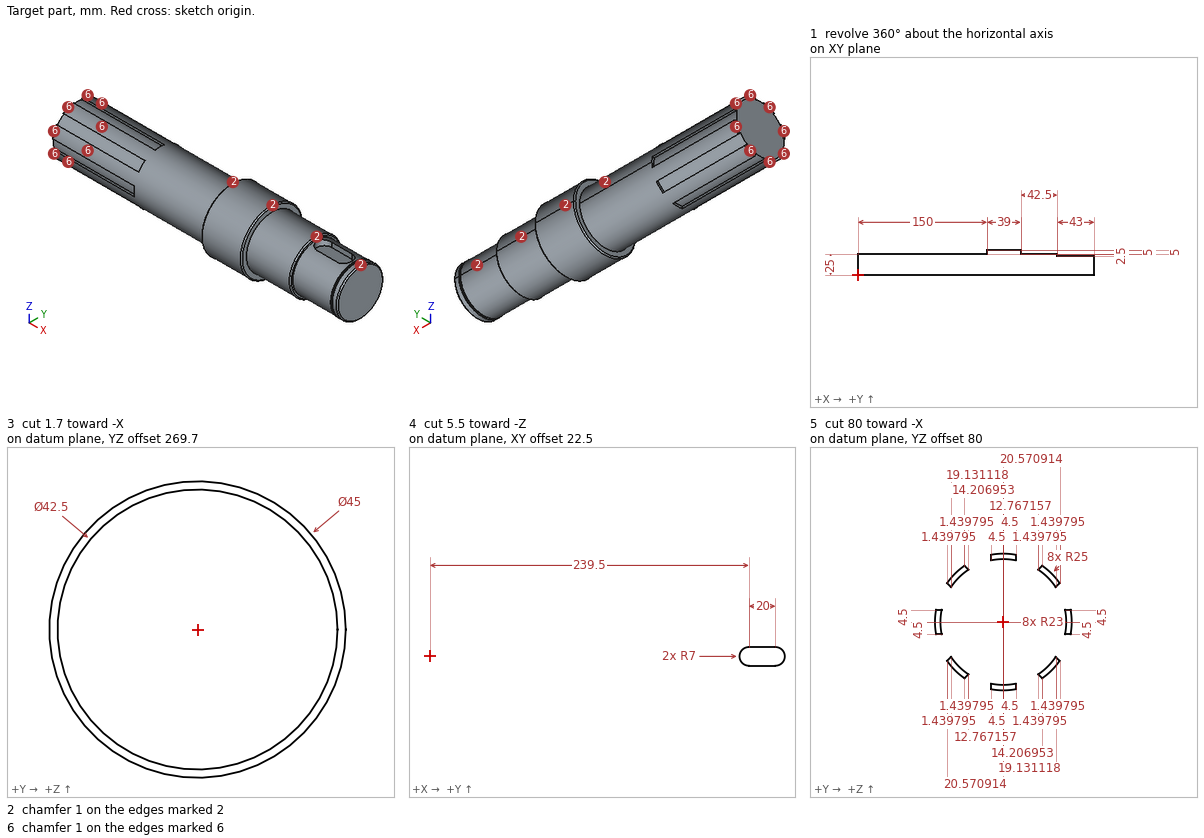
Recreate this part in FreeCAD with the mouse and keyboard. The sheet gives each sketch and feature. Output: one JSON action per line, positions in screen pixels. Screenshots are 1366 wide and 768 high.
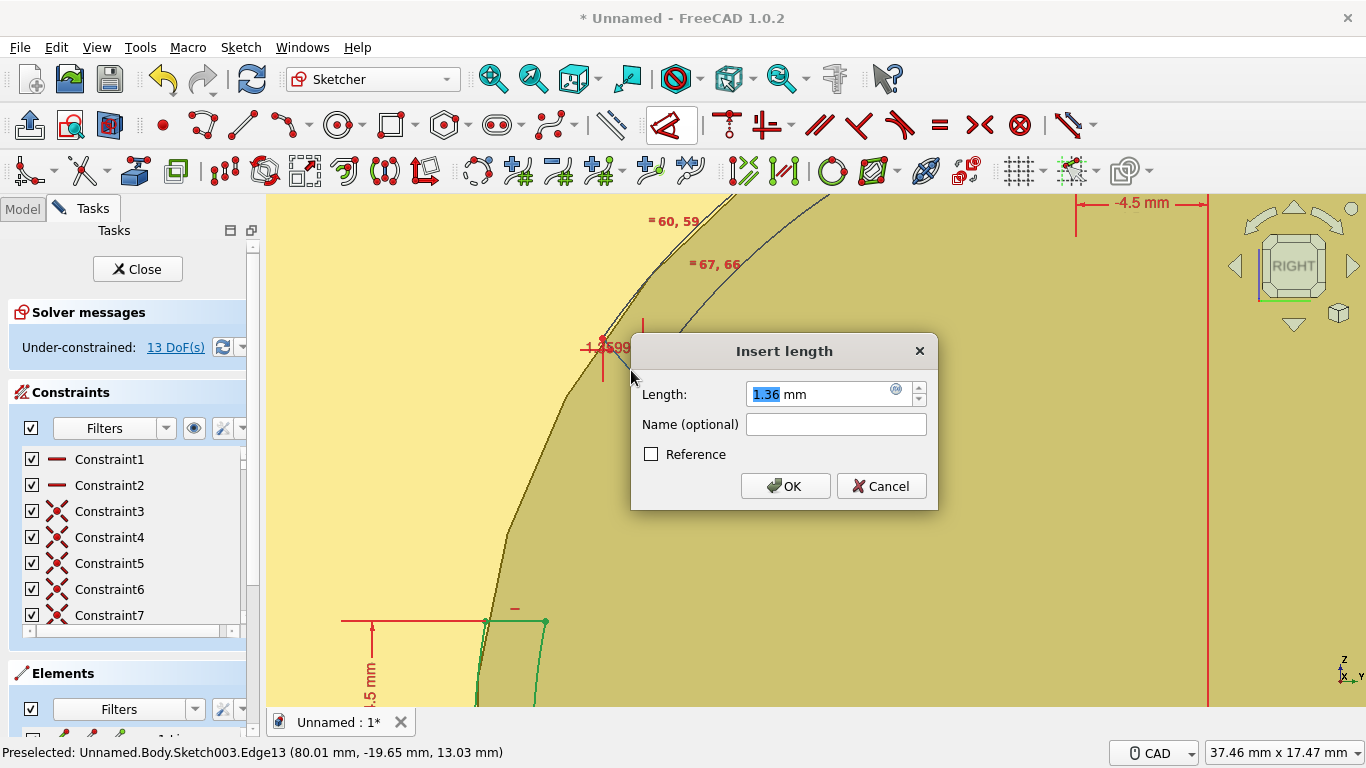
{"action": "type", "text": "1.439795"}
{"action": "key", "text": "Return"}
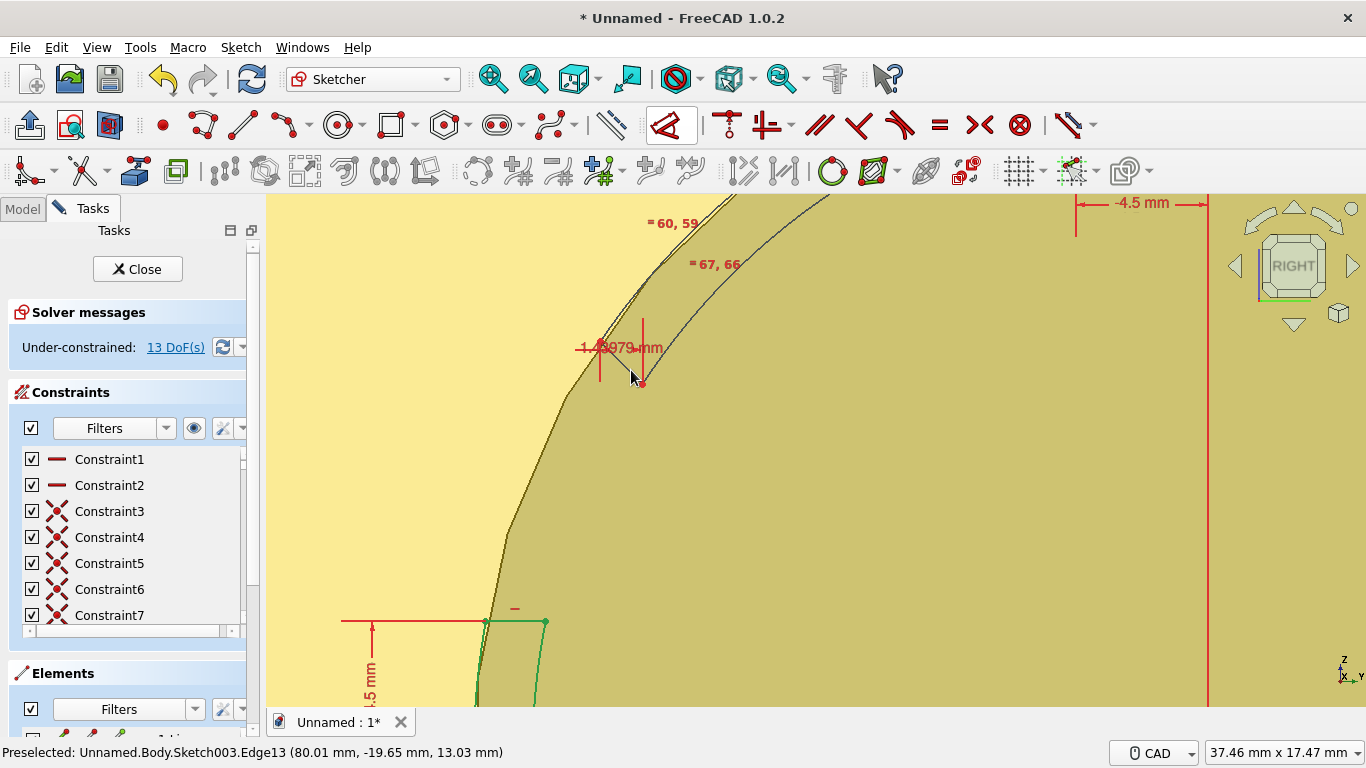
{"action": "scroll", "coordinate": [631, 374], "scroll_direction": "down", "scroll_amount": 8}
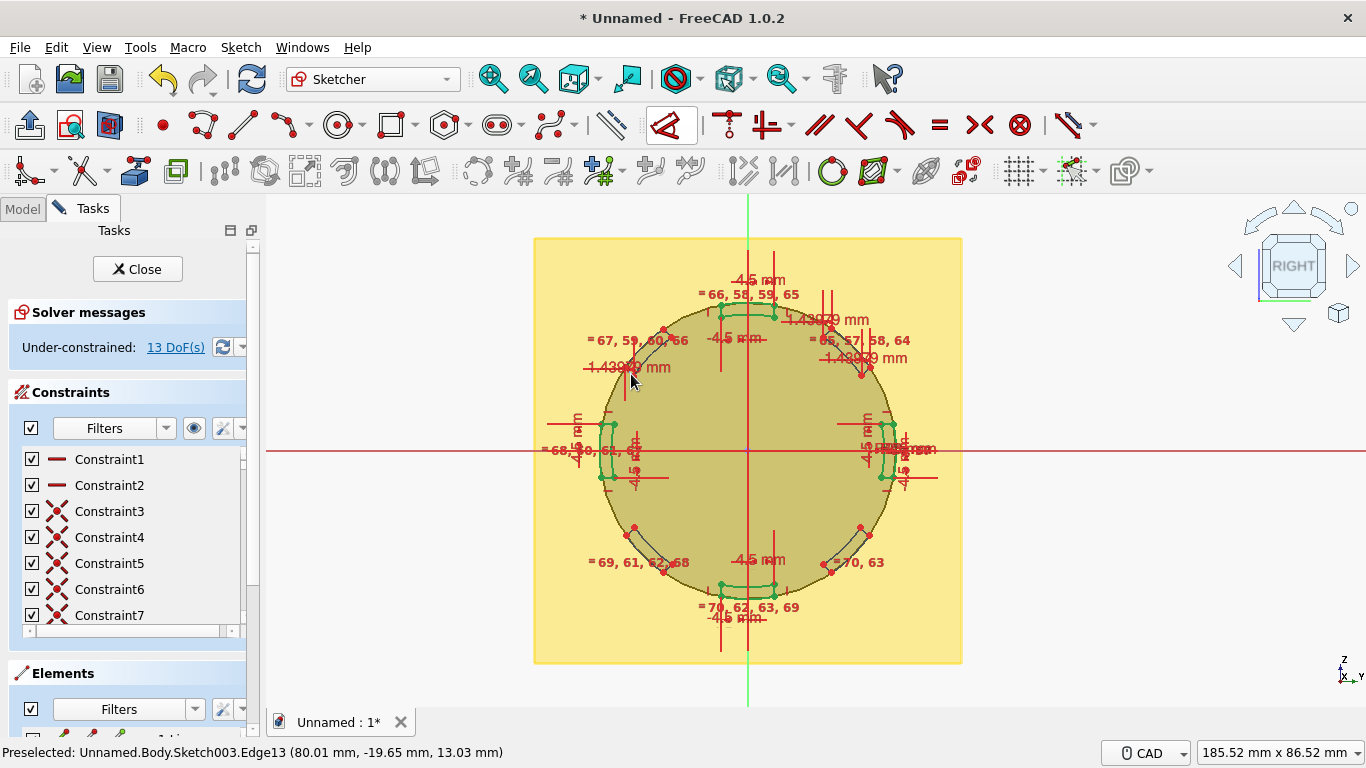
{"action": "scroll", "coordinate": [666, 332], "scroll_direction": "up", "scroll_amount": 8}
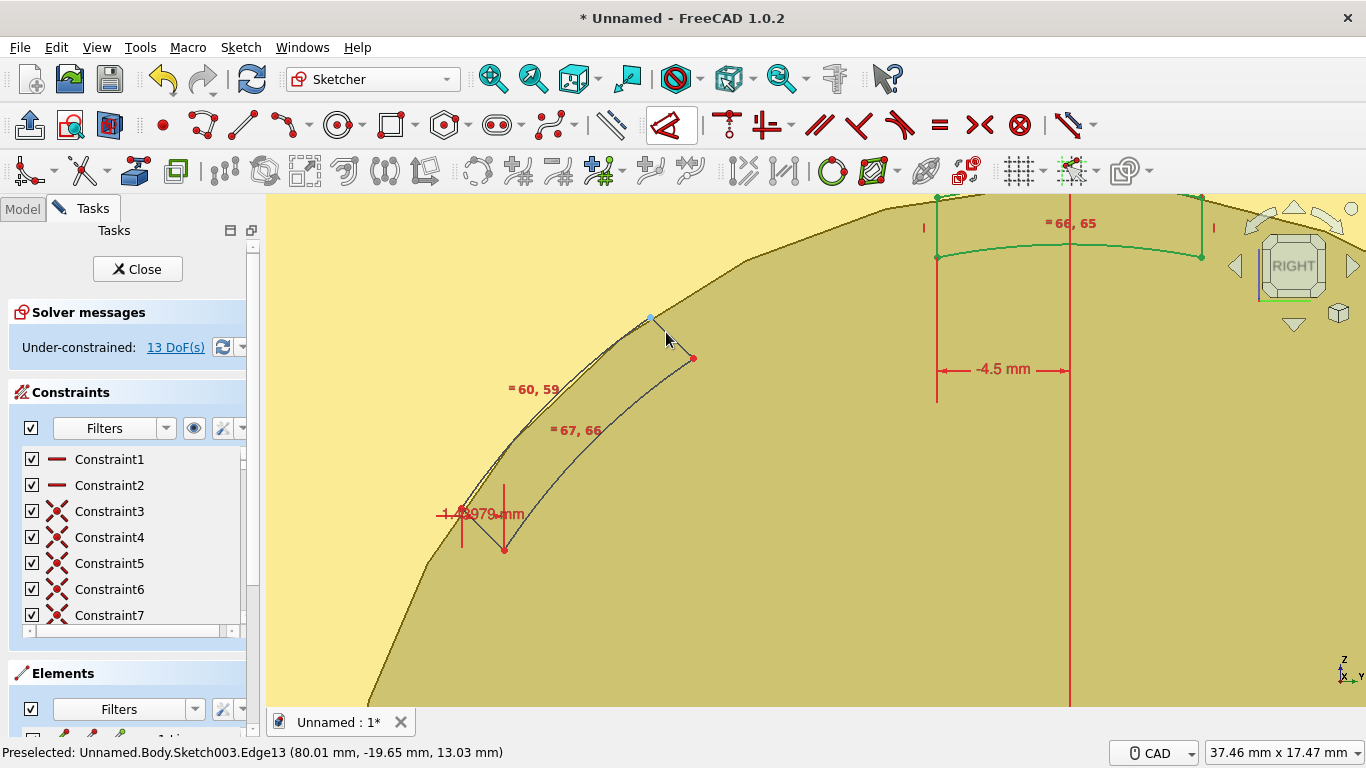
{"action": "left_click", "coordinate": [663, 330]}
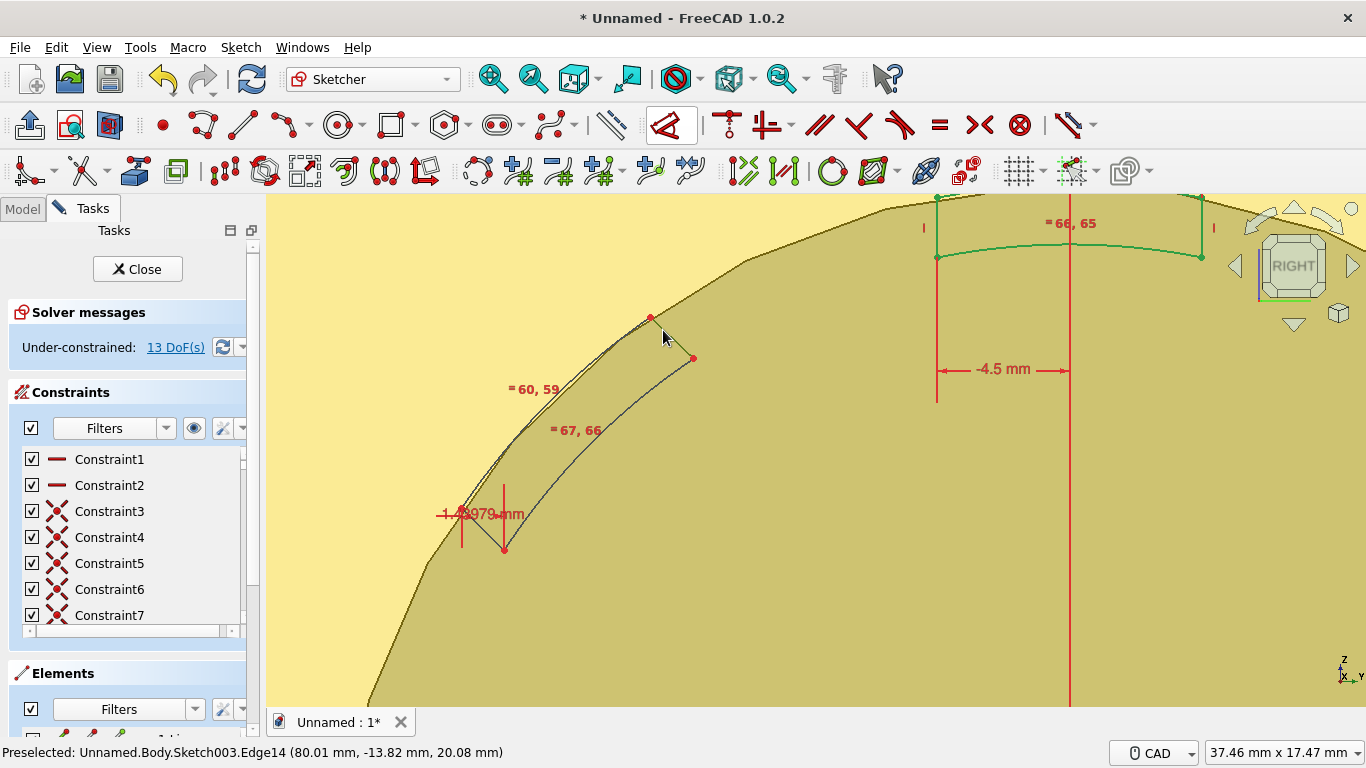
{"action": "key", "text": "l"}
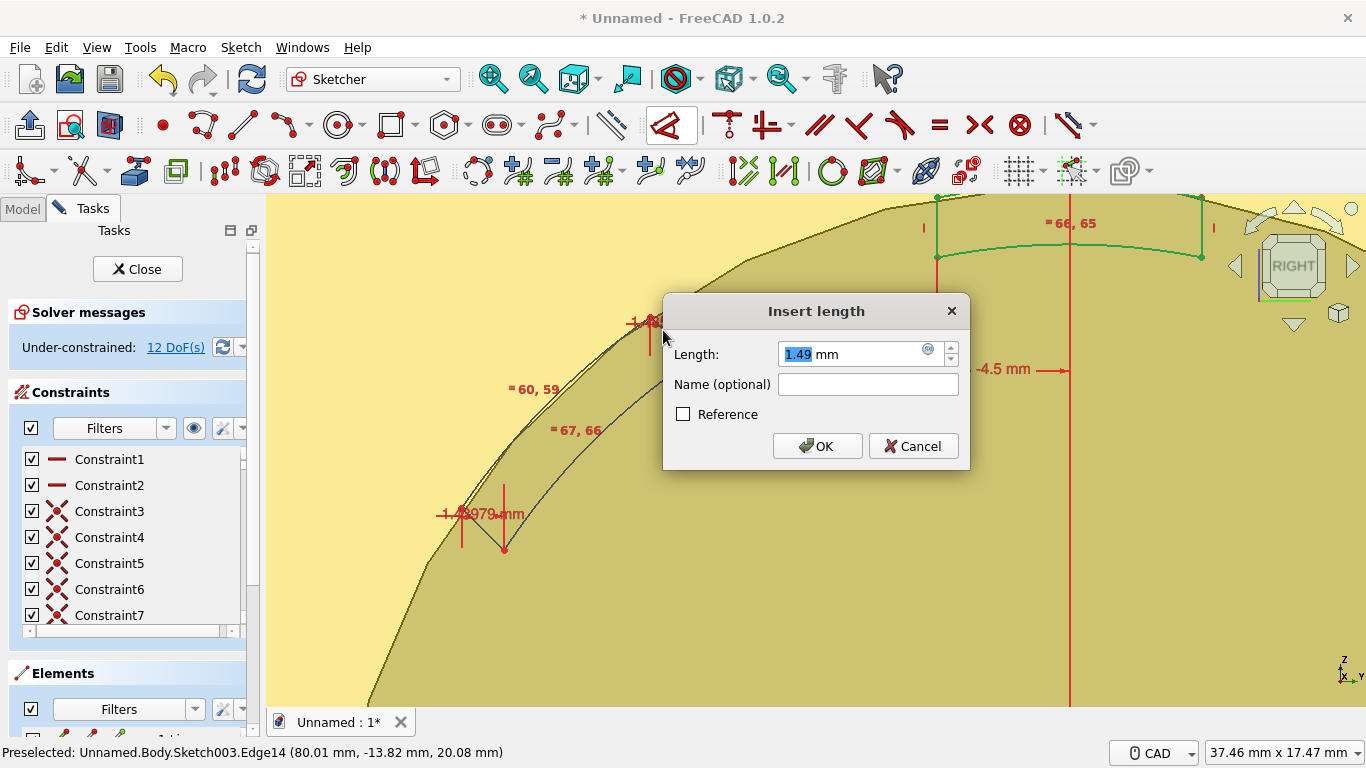
{"action": "type", "text": "1.439795"}
{"action": "key", "text": "Return"}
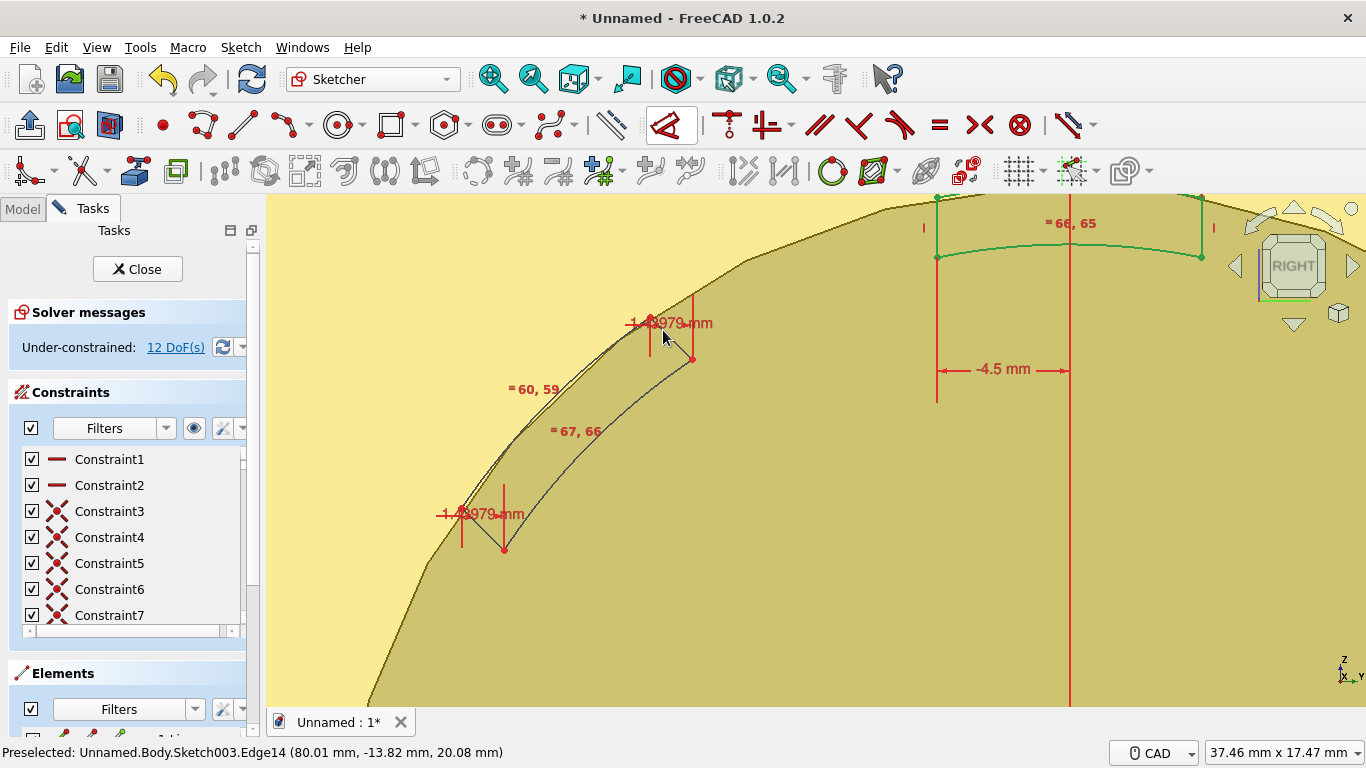
{"action": "scroll", "coordinate": [666, 332], "scroll_direction": "down", "scroll_amount": 8}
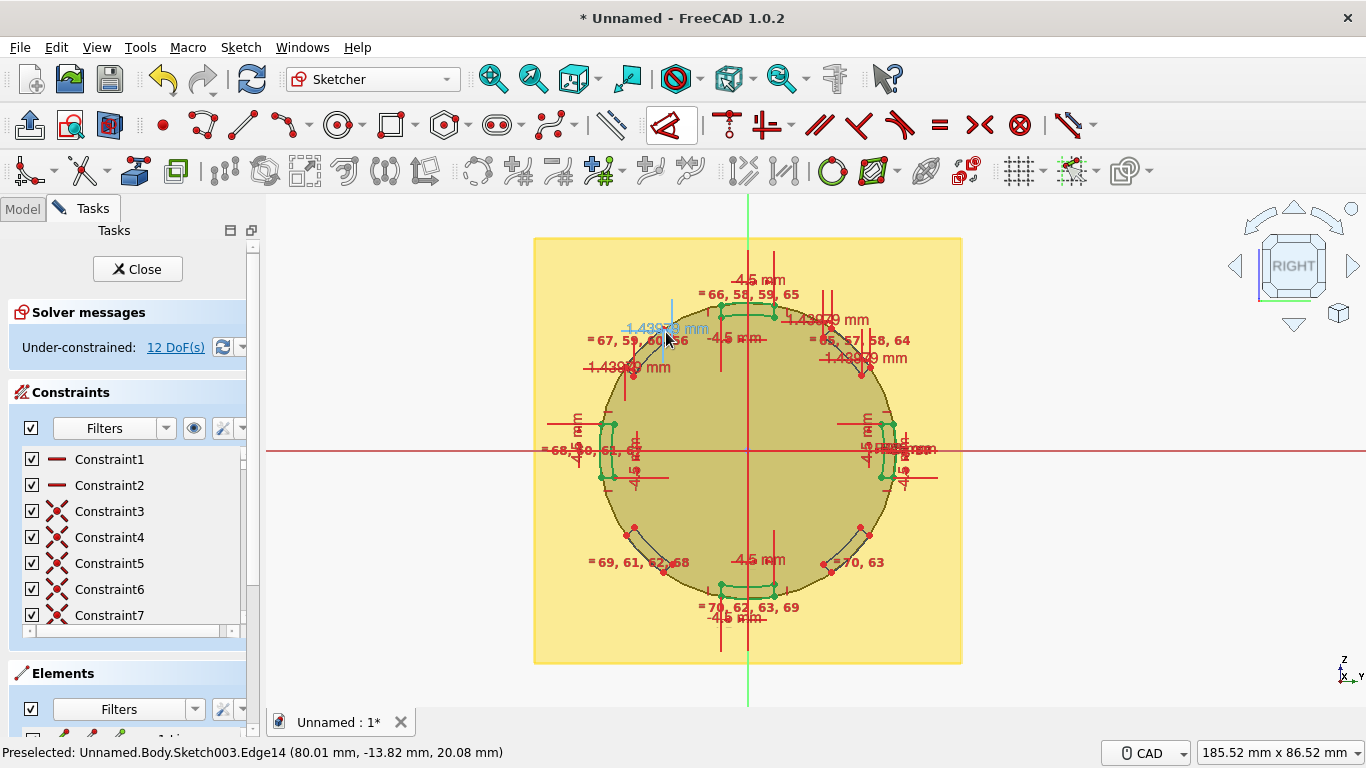
{"action": "scroll", "coordinate": [669, 567], "scroll_direction": "up", "scroll_amount": 8}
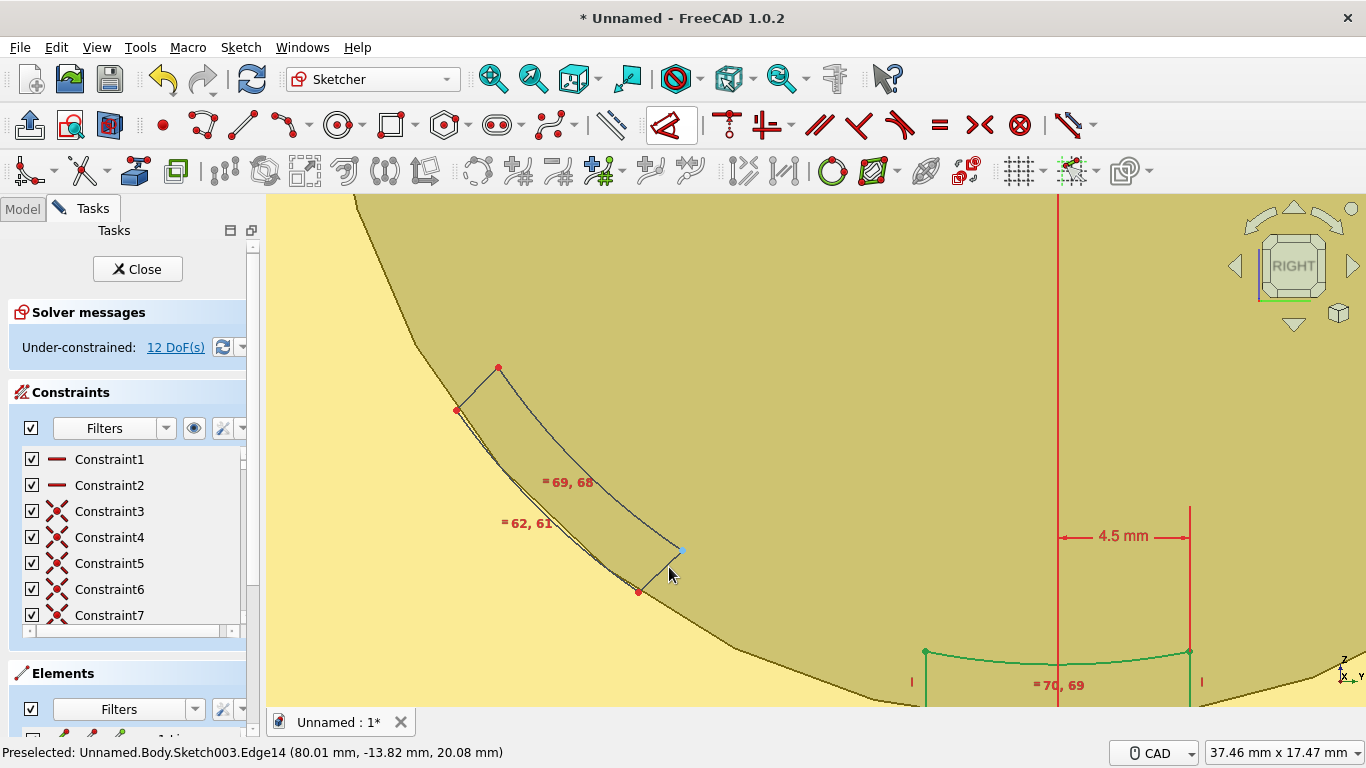
{"action": "left_click", "coordinate": [669, 563]}